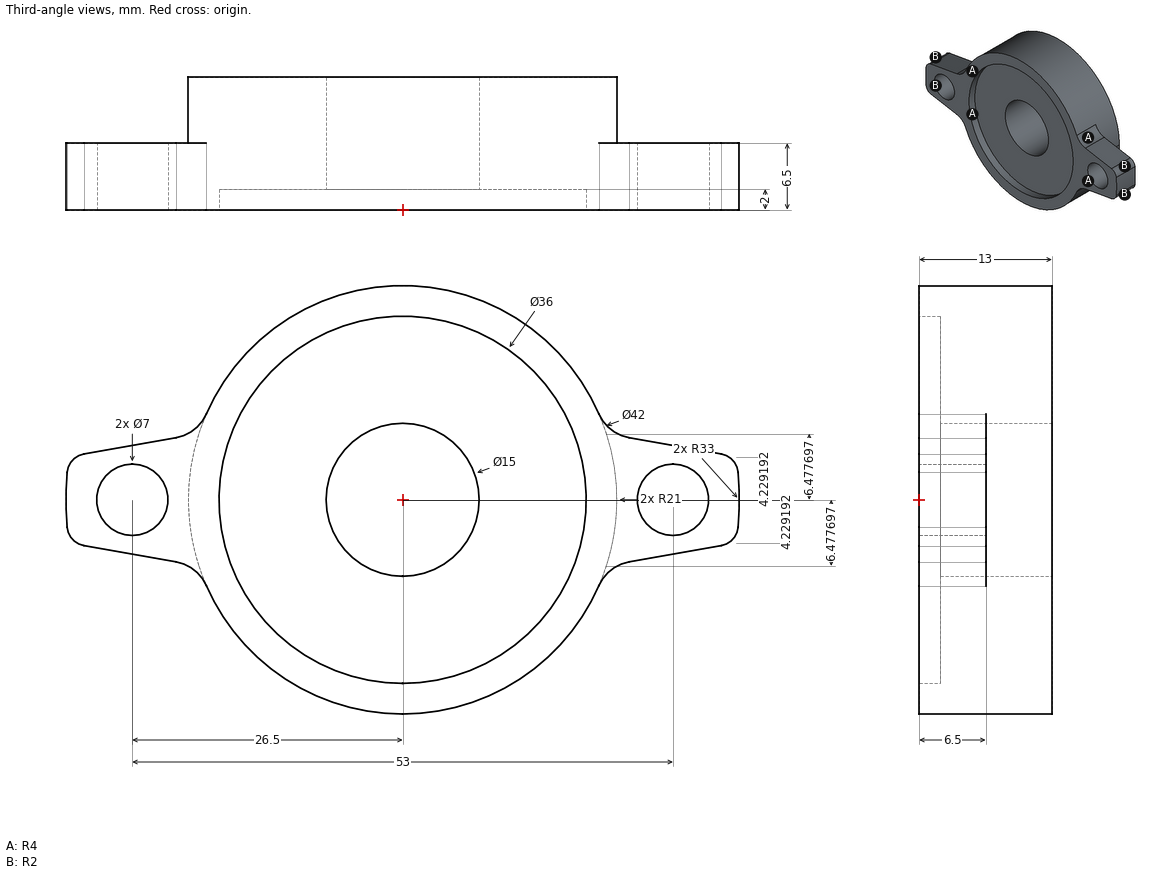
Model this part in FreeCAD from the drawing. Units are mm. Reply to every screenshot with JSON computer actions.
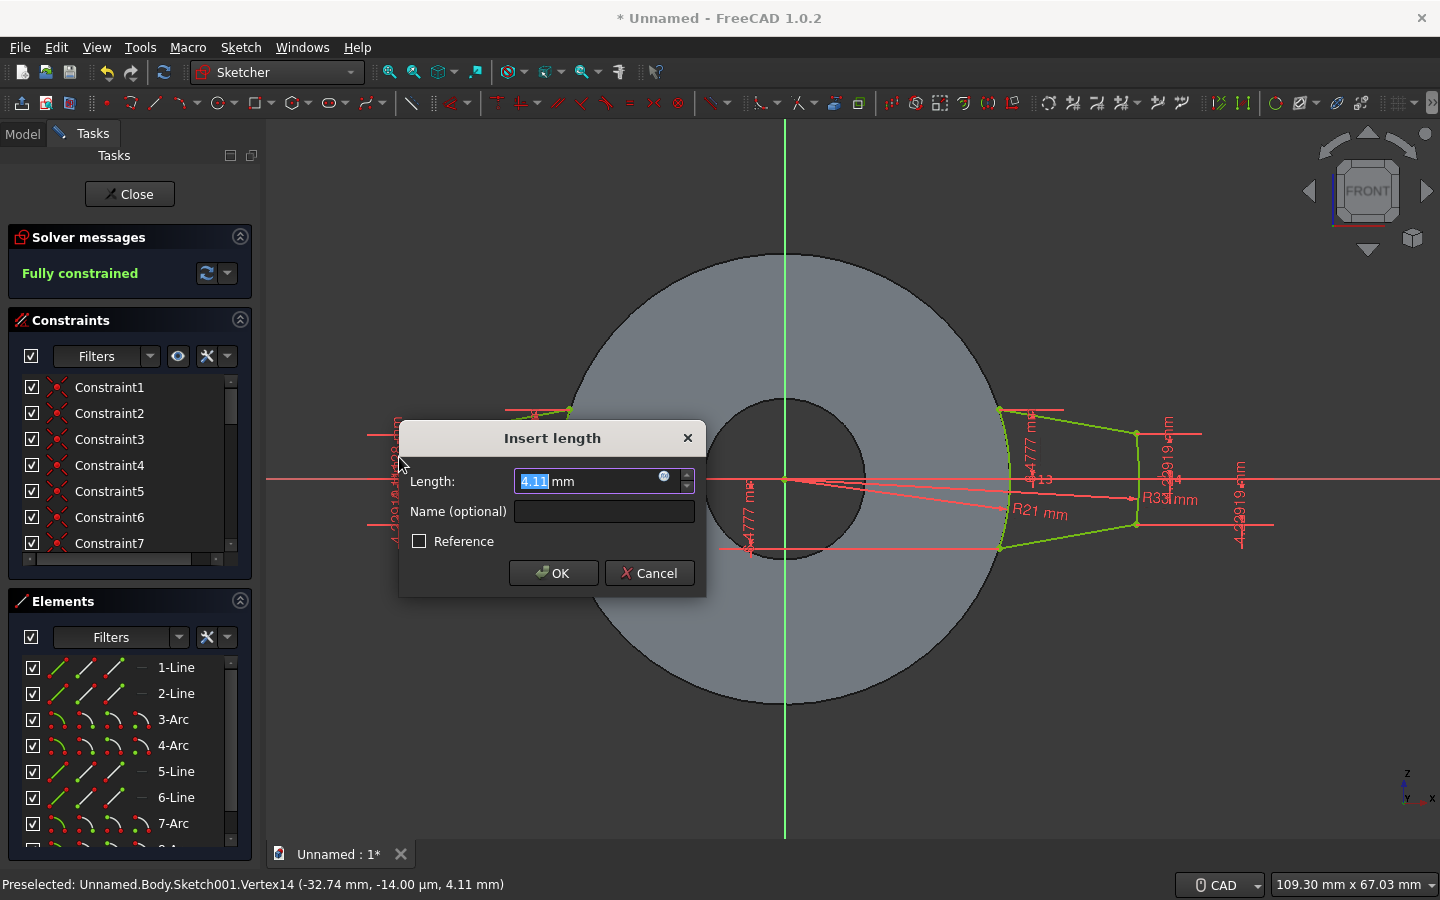
{"action": "type", "text": "4.229192"}
{"action": "key", "text": "Return"}
{"action": "key", "text": "Escape"}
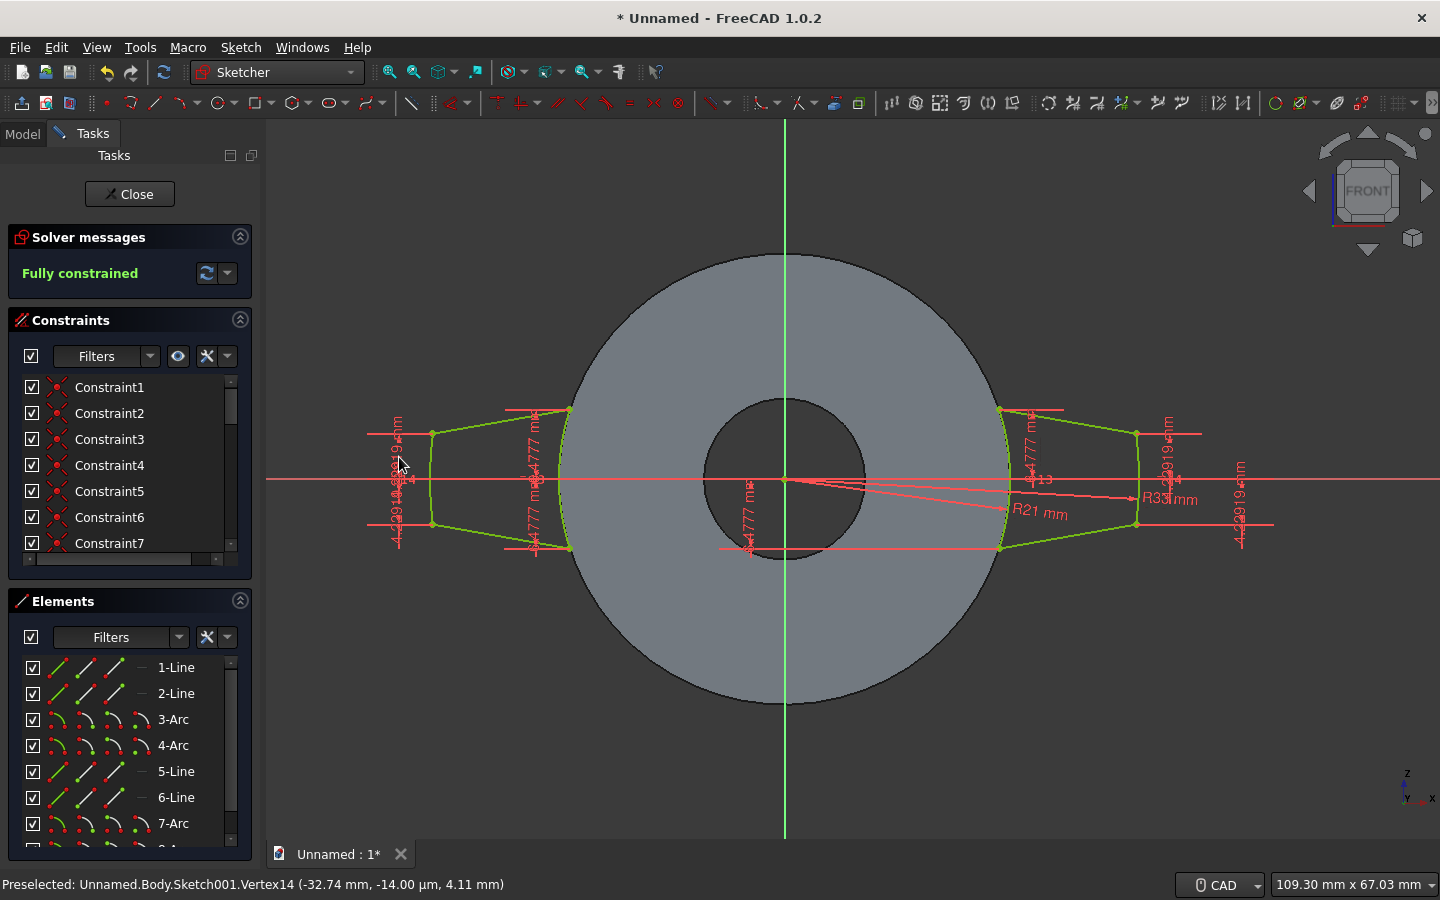
{"action": "left_click", "coordinate": [130, 194]}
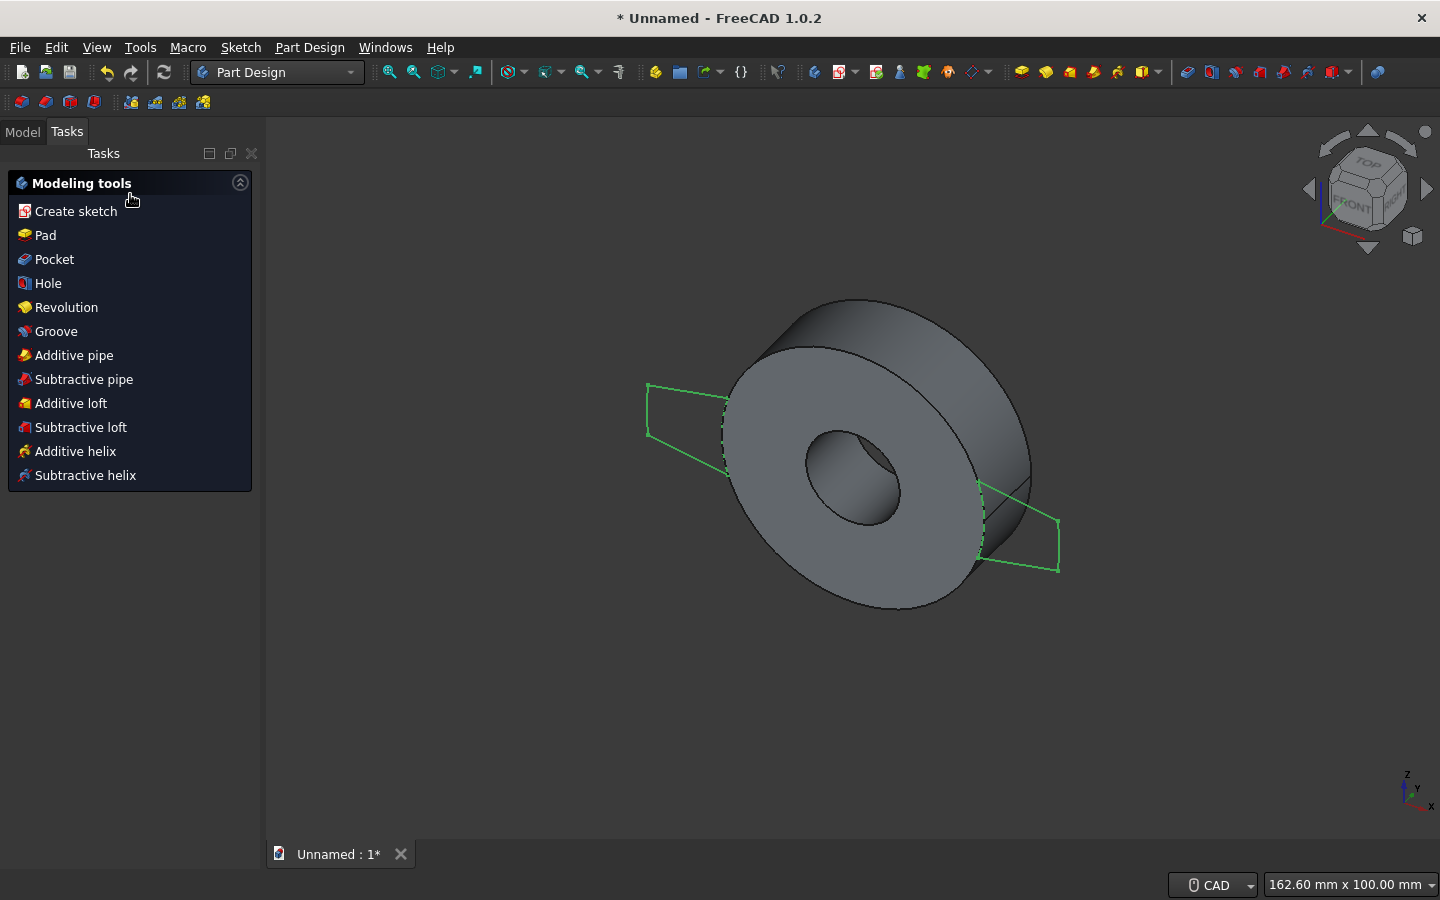
{"action": "left_click", "coordinate": [1022, 72]}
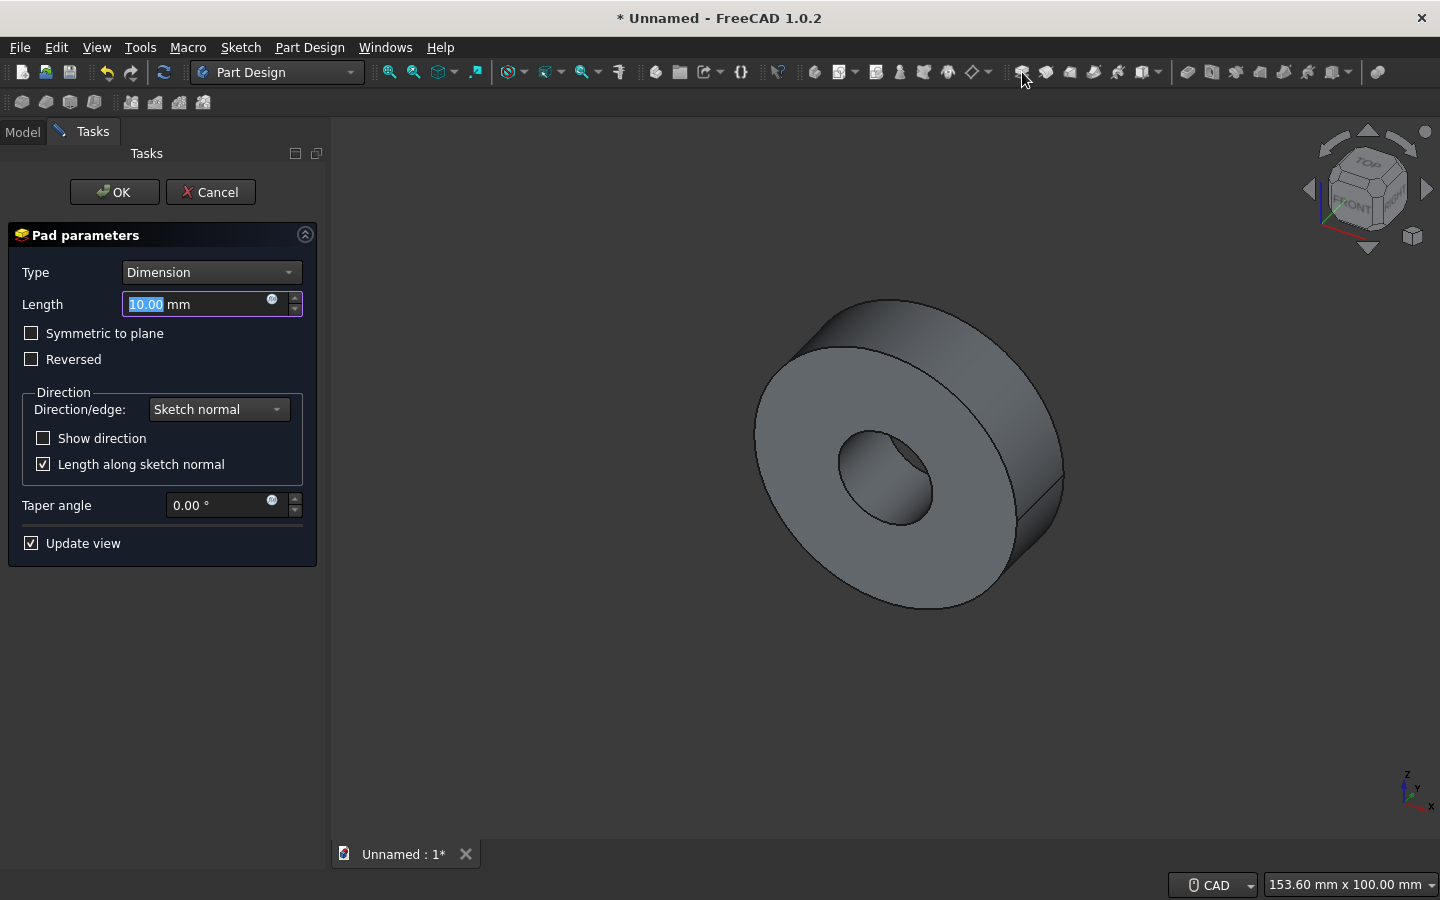
{"action": "type", "text": "6.5"}
{"action": "key", "text": "Tab"}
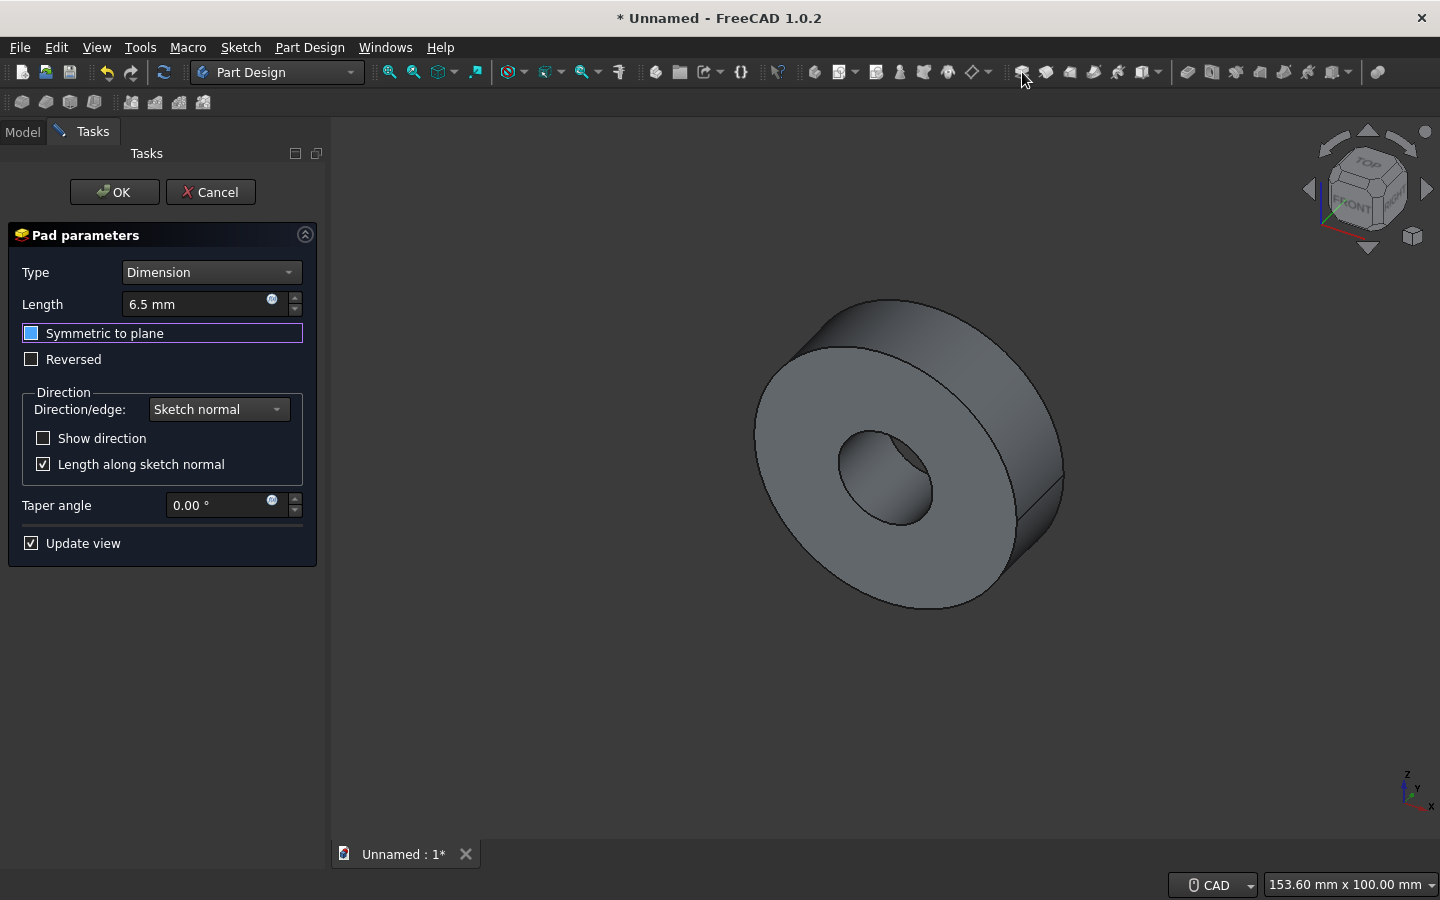
{"action": "left_click", "coordinate": [30, 359]}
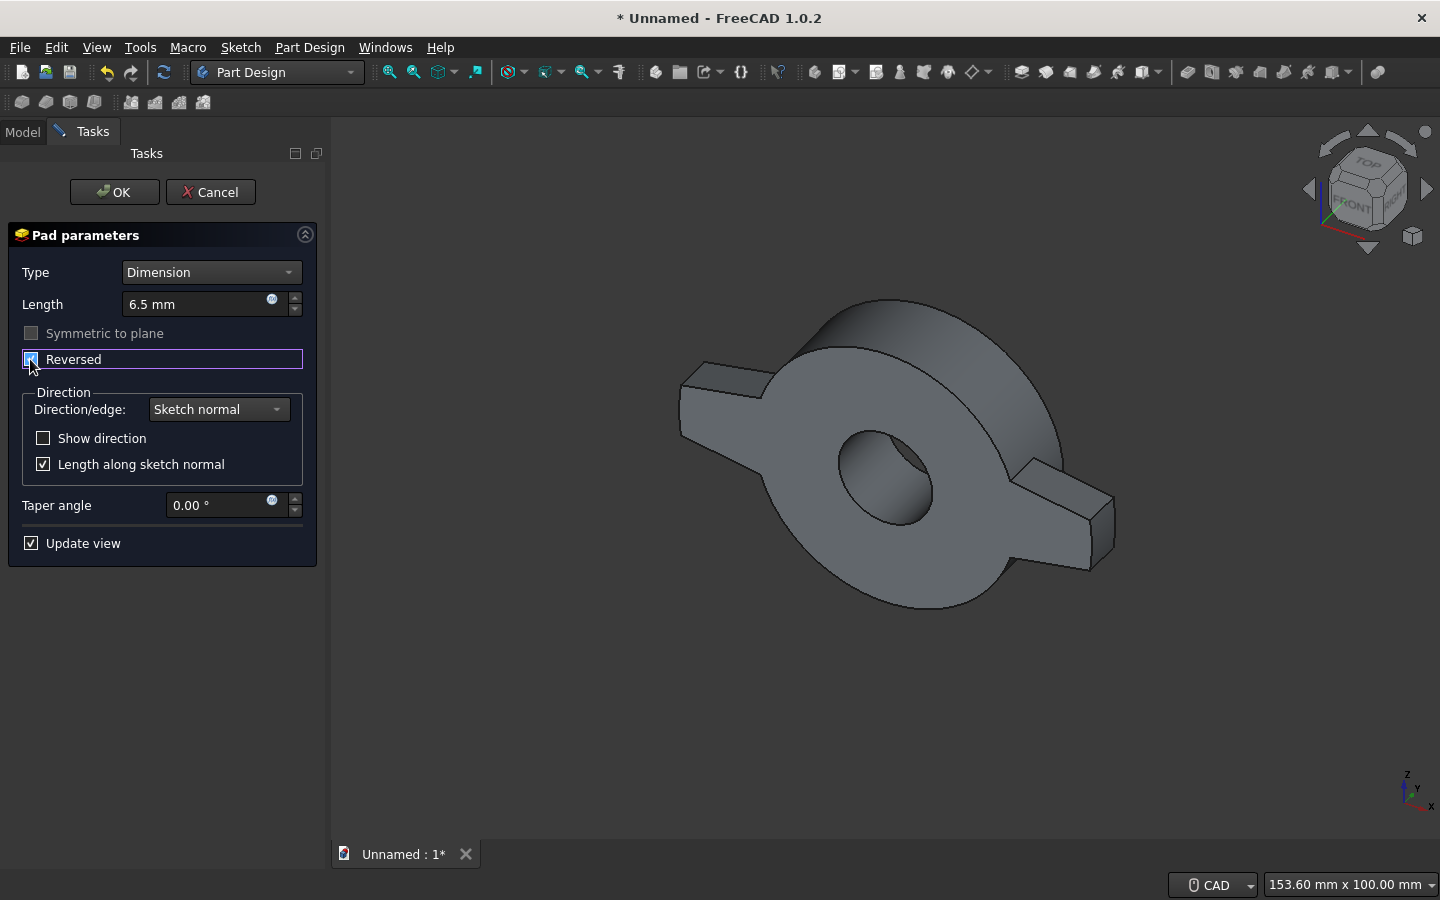
{"action": "left_click", "coordinate": [115, 192]}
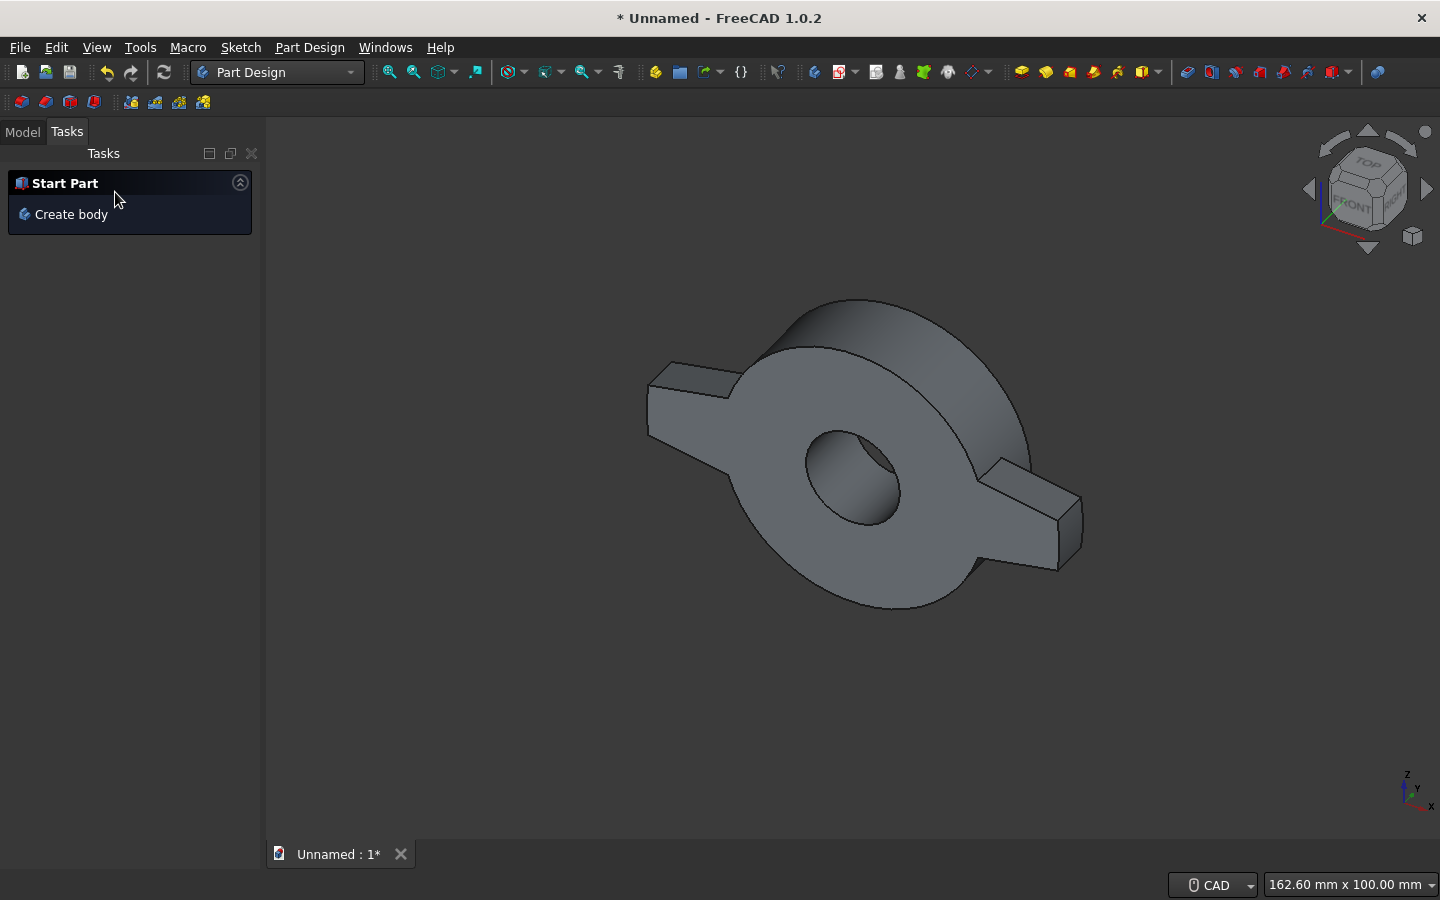
{"action": "key", "text": "0"}